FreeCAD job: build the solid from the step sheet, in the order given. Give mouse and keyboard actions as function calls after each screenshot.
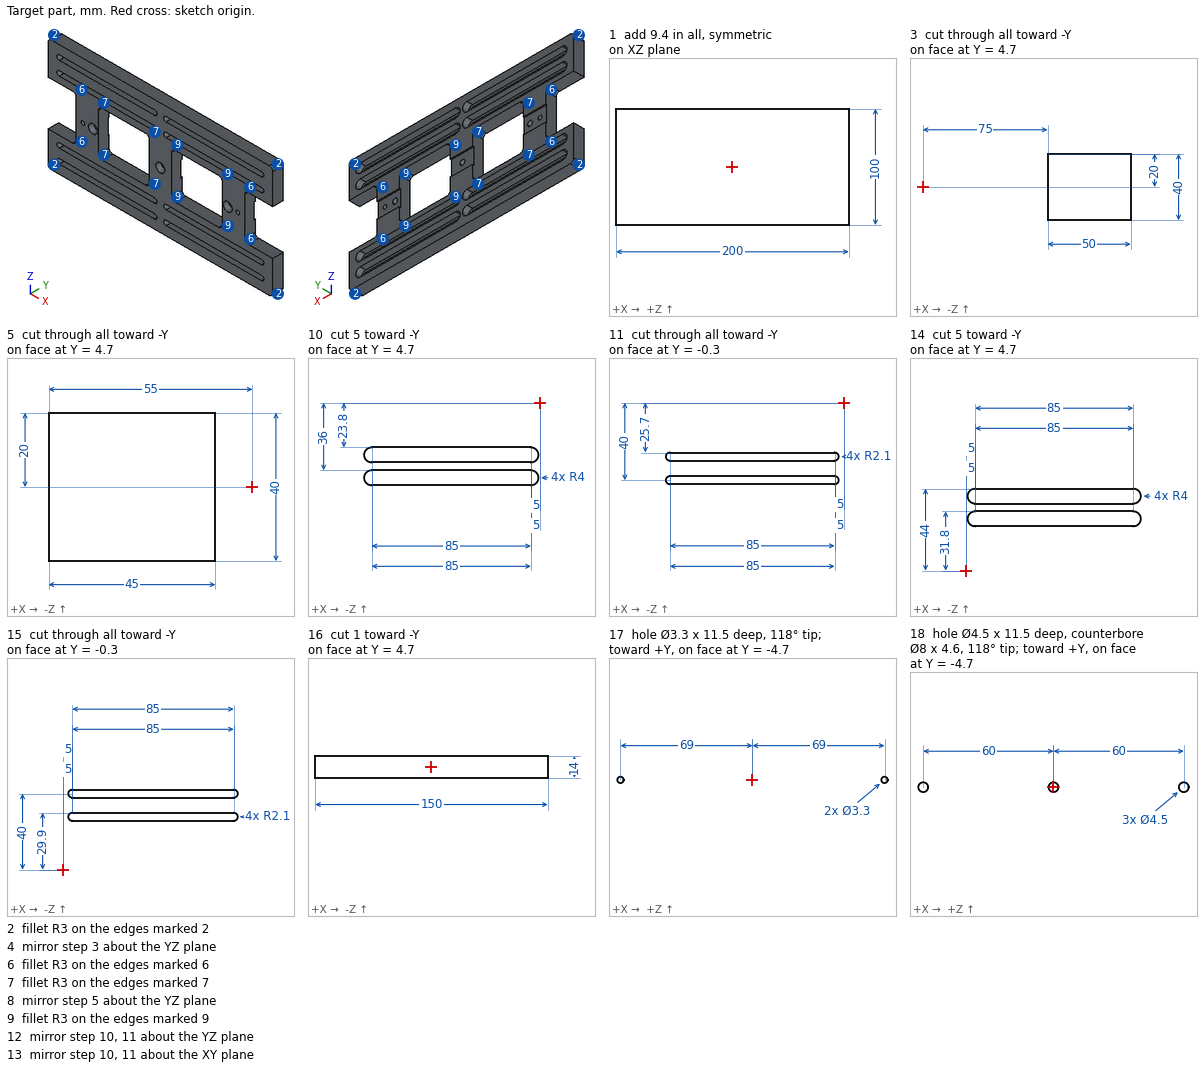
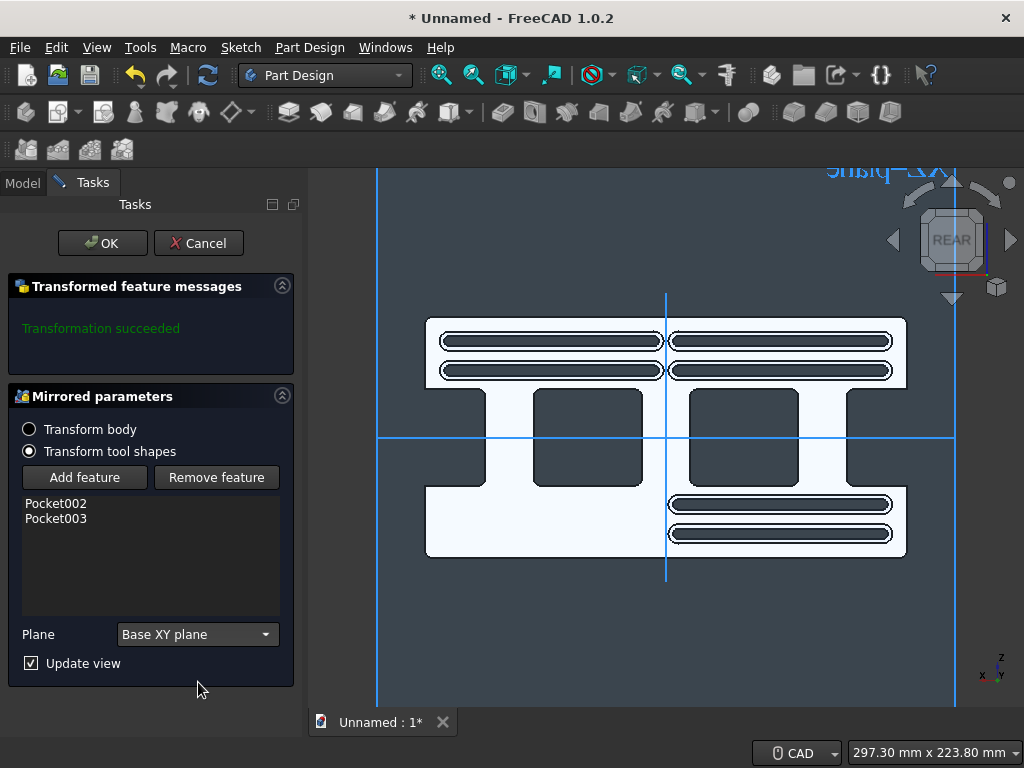
click(103, 243)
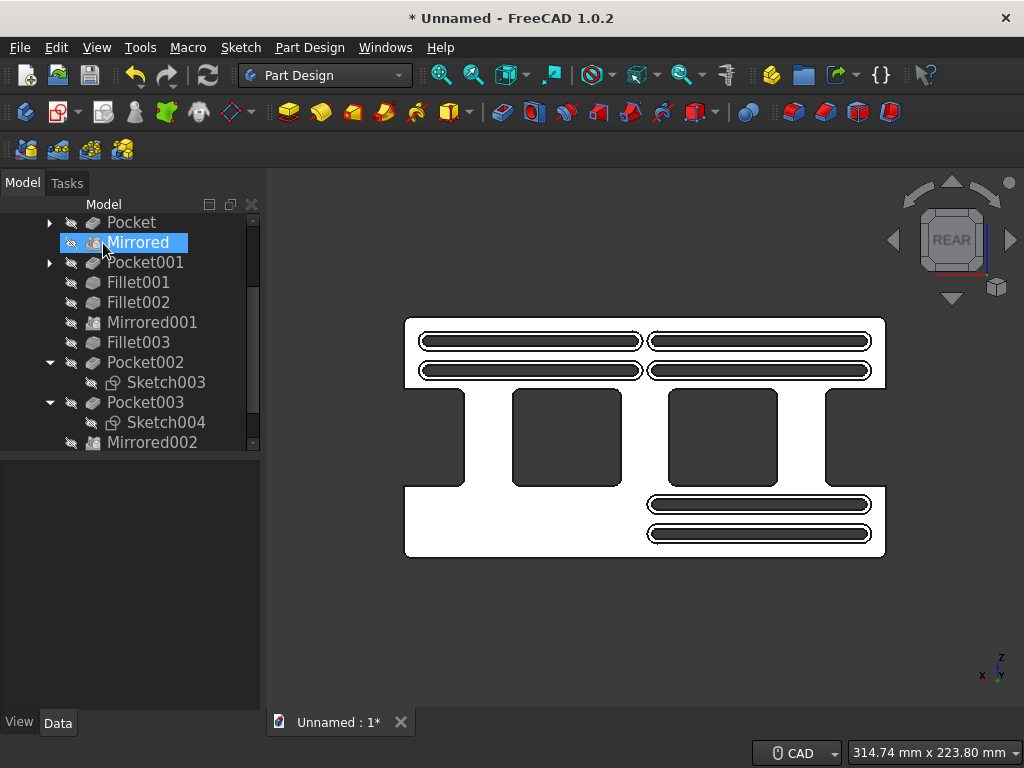
click(645, 437)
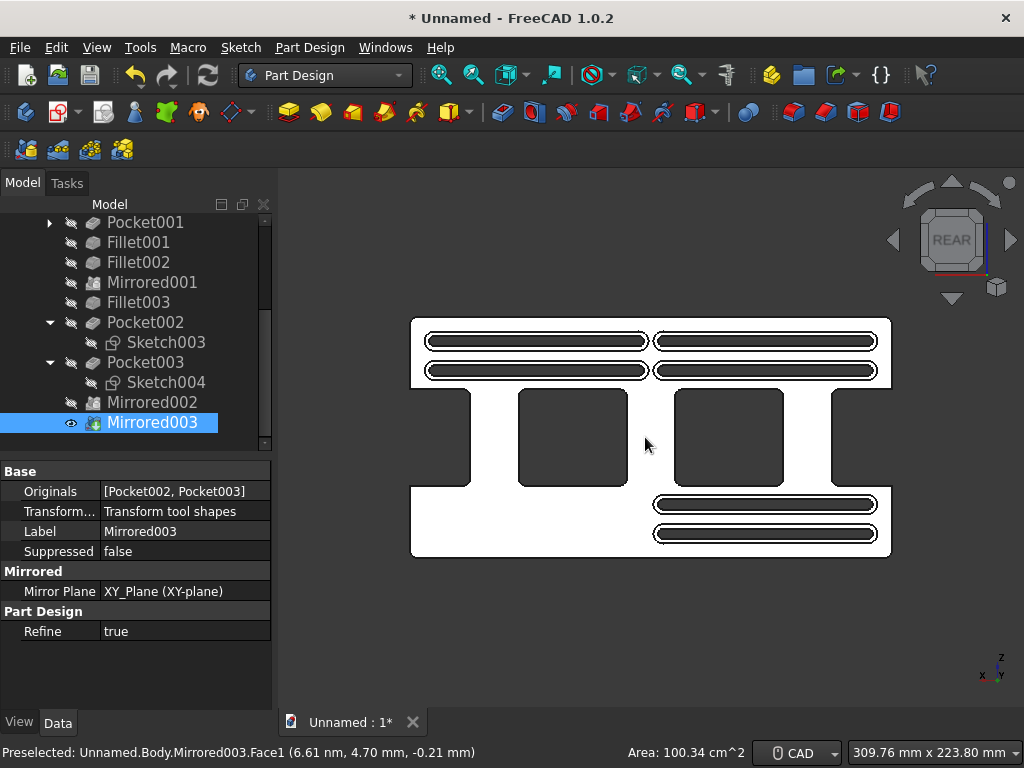
click(58, 112)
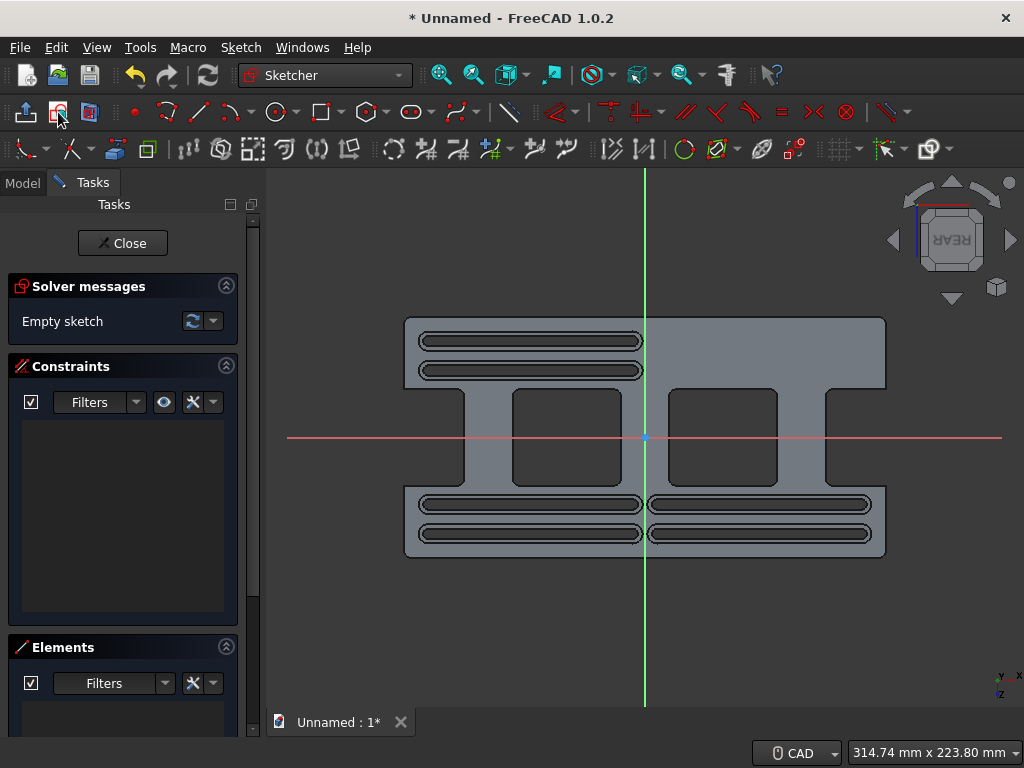
scroll(576, 438, down, 5)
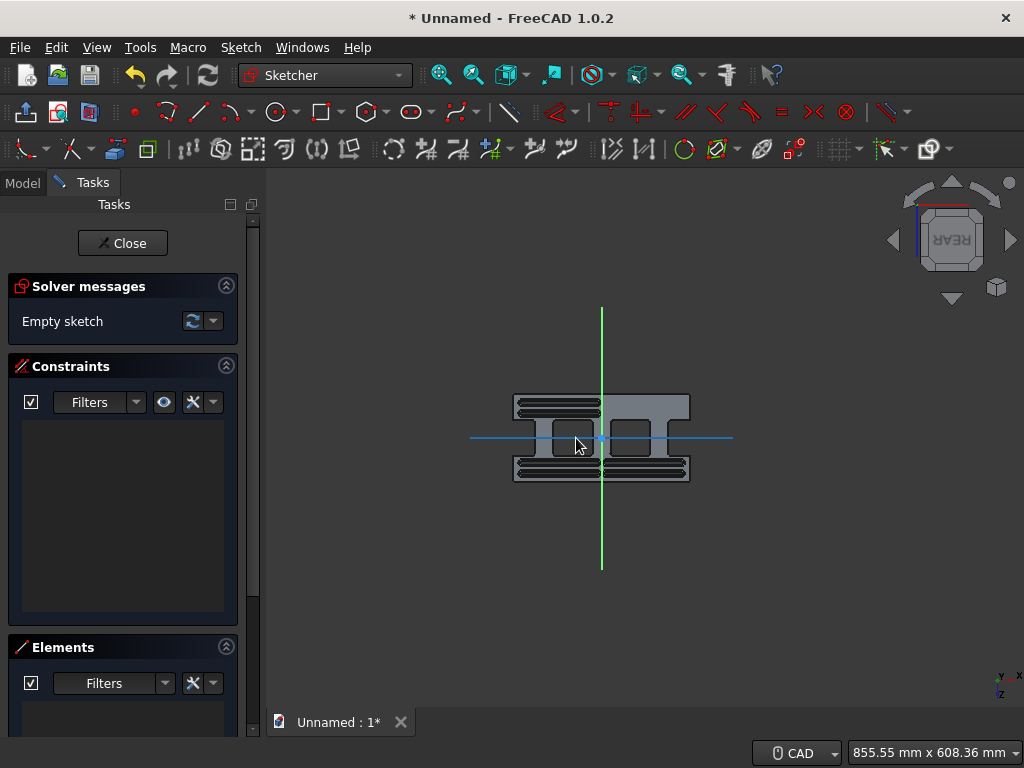
scroll(660, 414, up, 8)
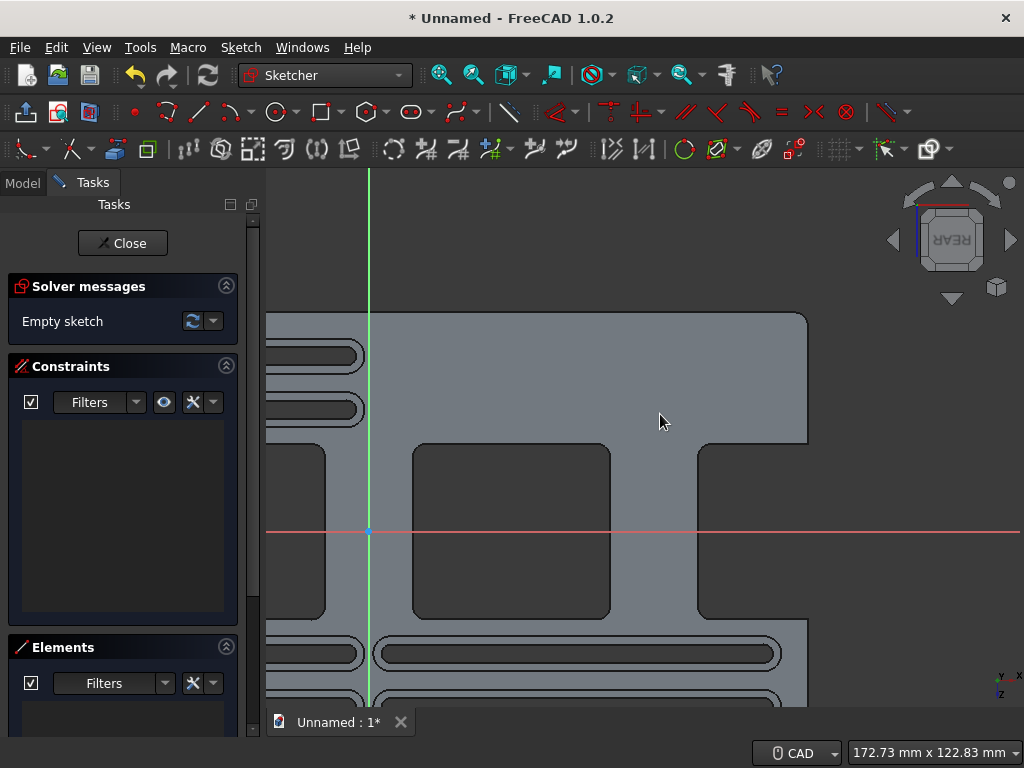
click(412, 112)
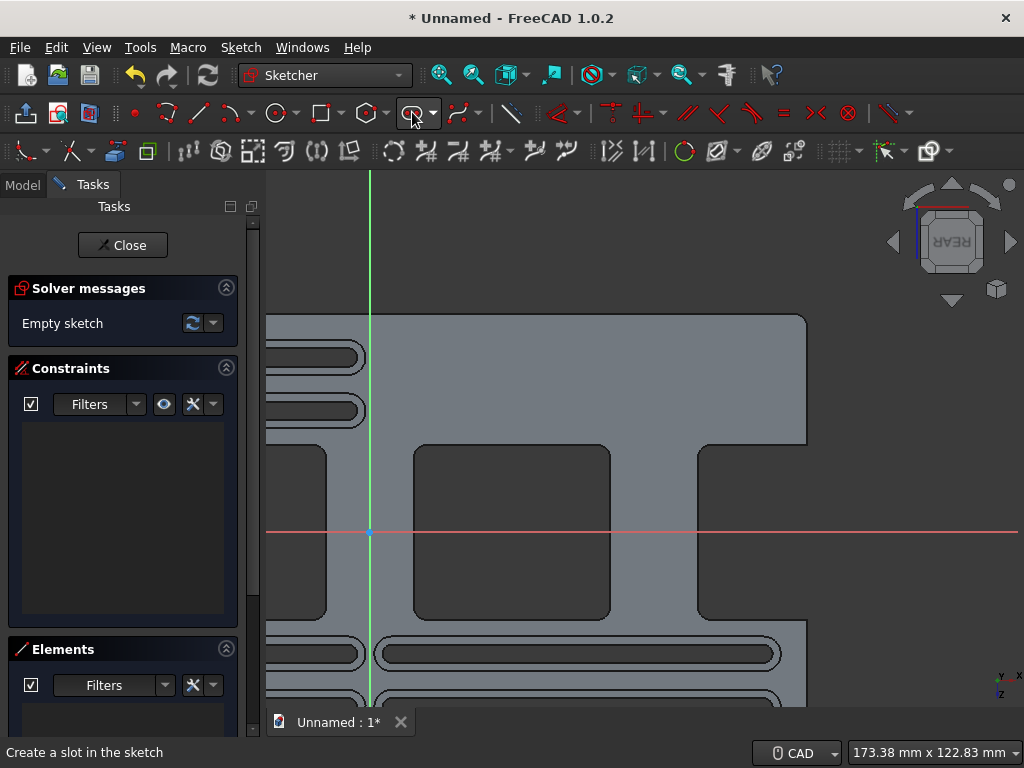
scroll(392, 357, up, 2)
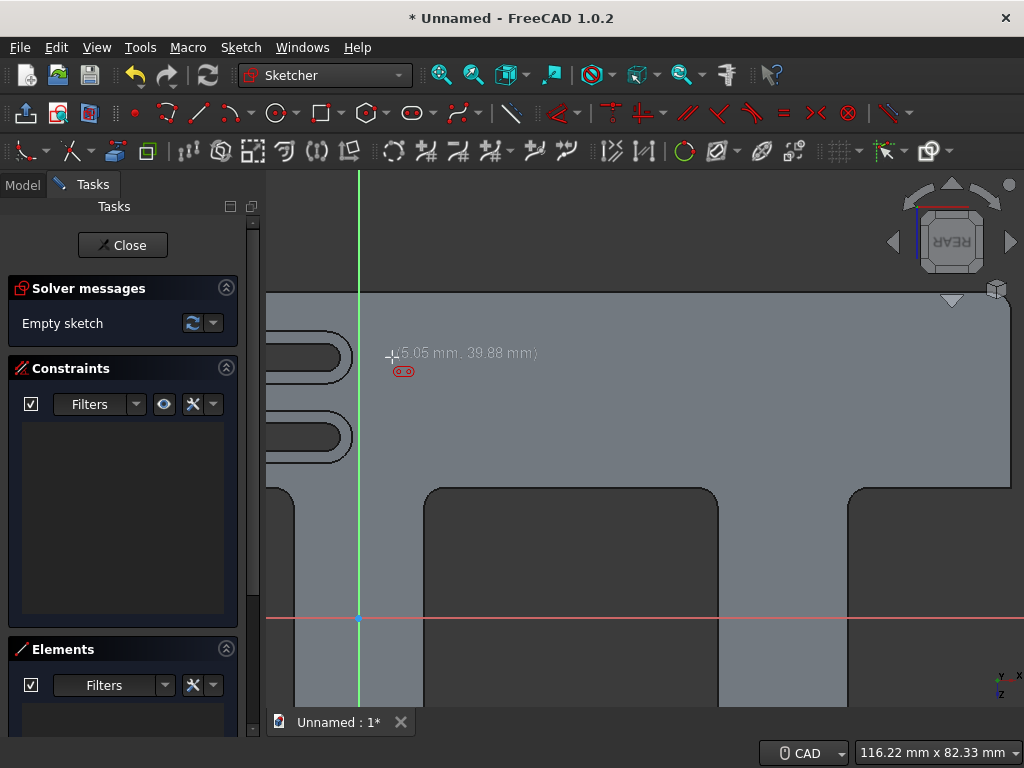
click(392, 358)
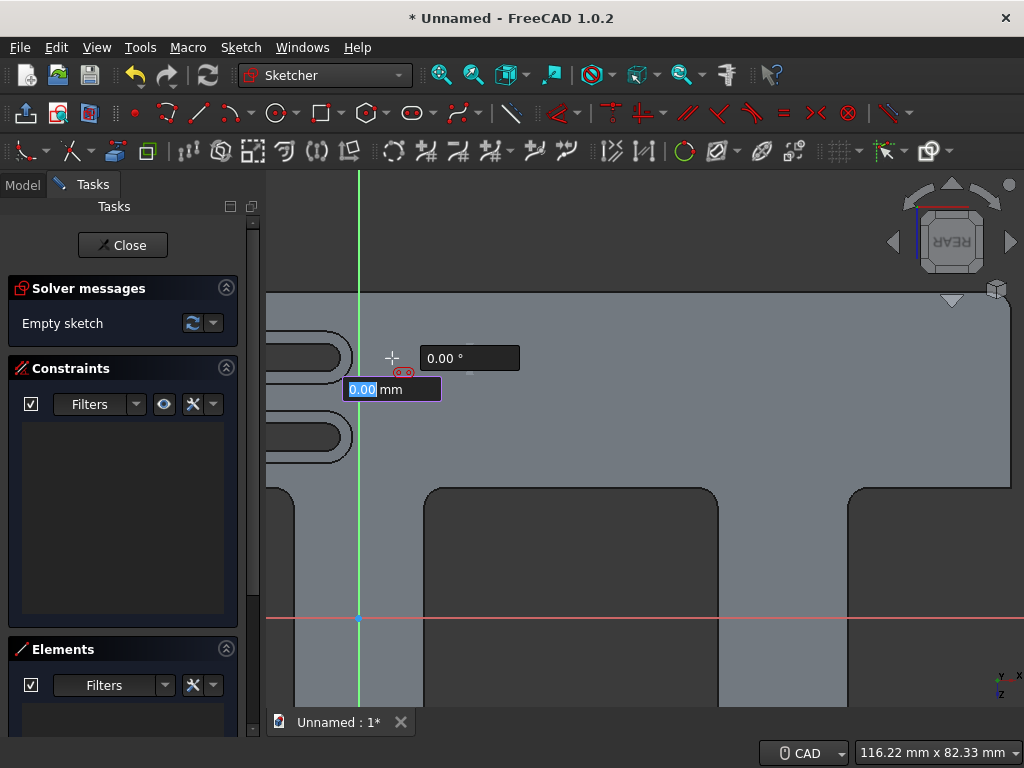
scroll(395, 364, down, 2)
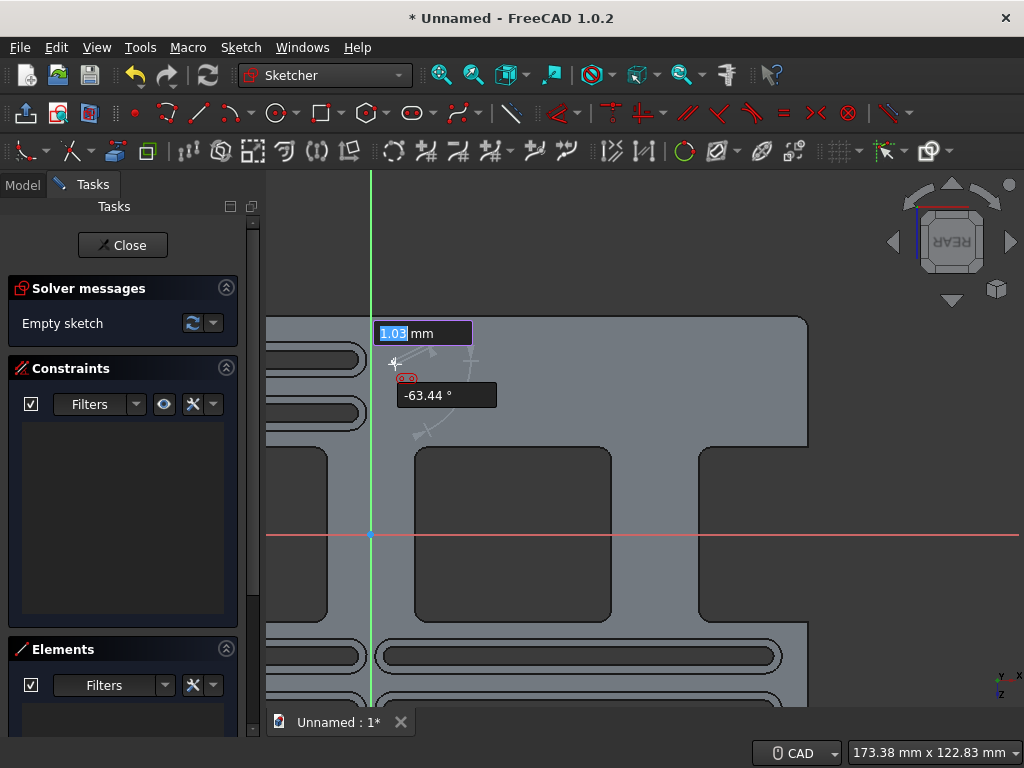
click(764, 360)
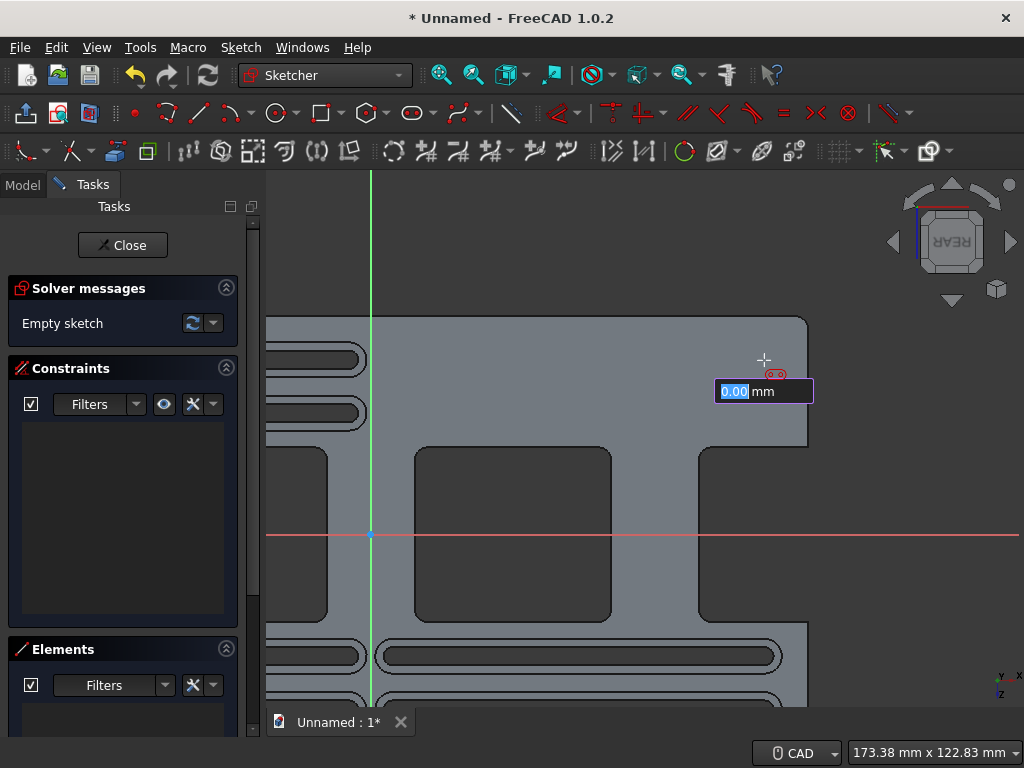
click(579, 377)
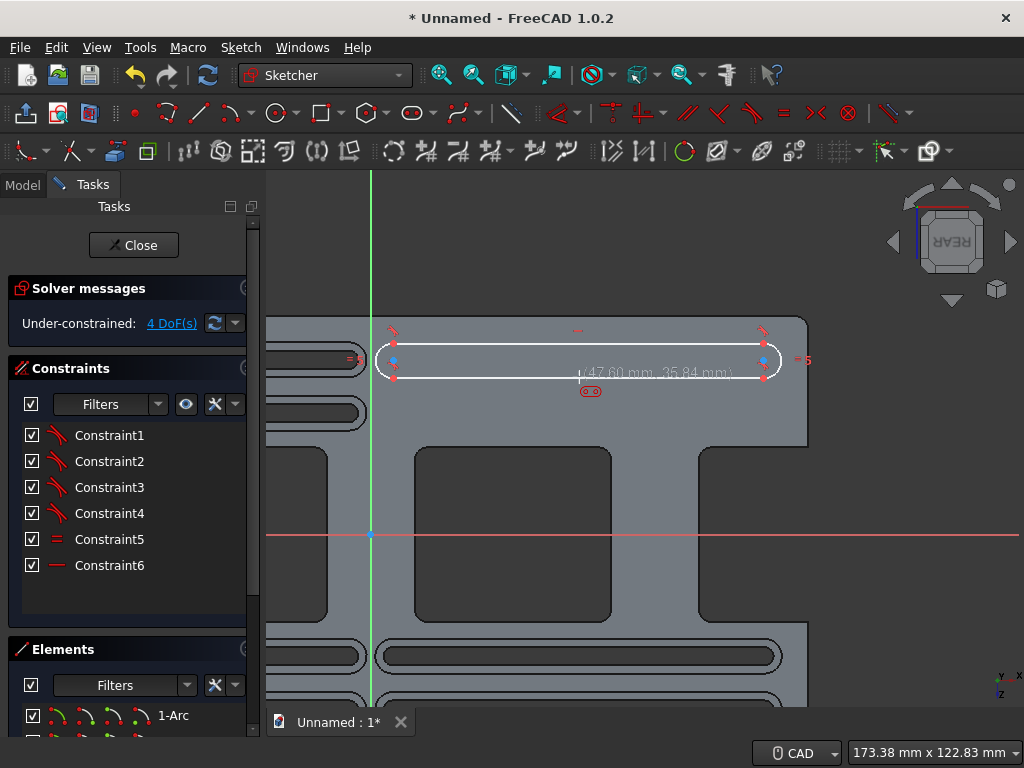
scroll(393, 413, up, 2)